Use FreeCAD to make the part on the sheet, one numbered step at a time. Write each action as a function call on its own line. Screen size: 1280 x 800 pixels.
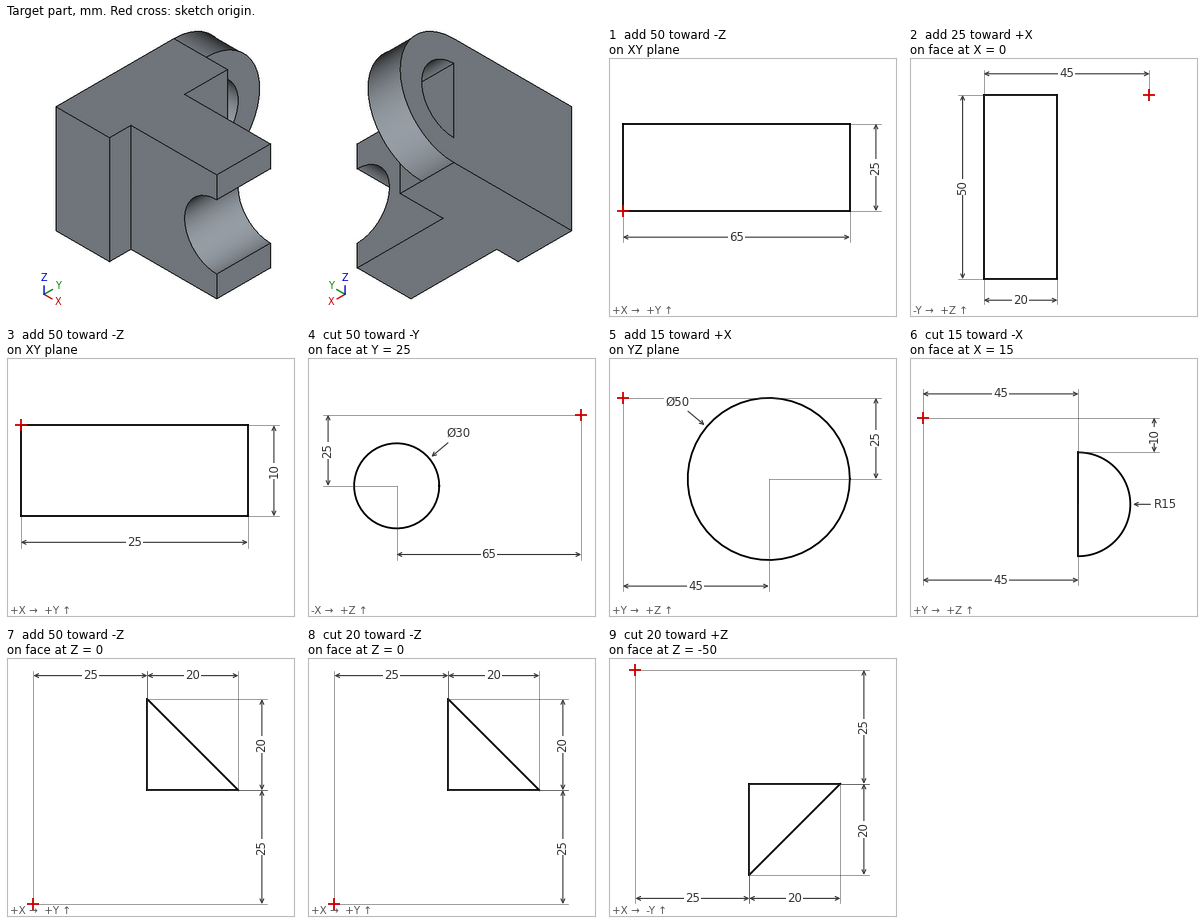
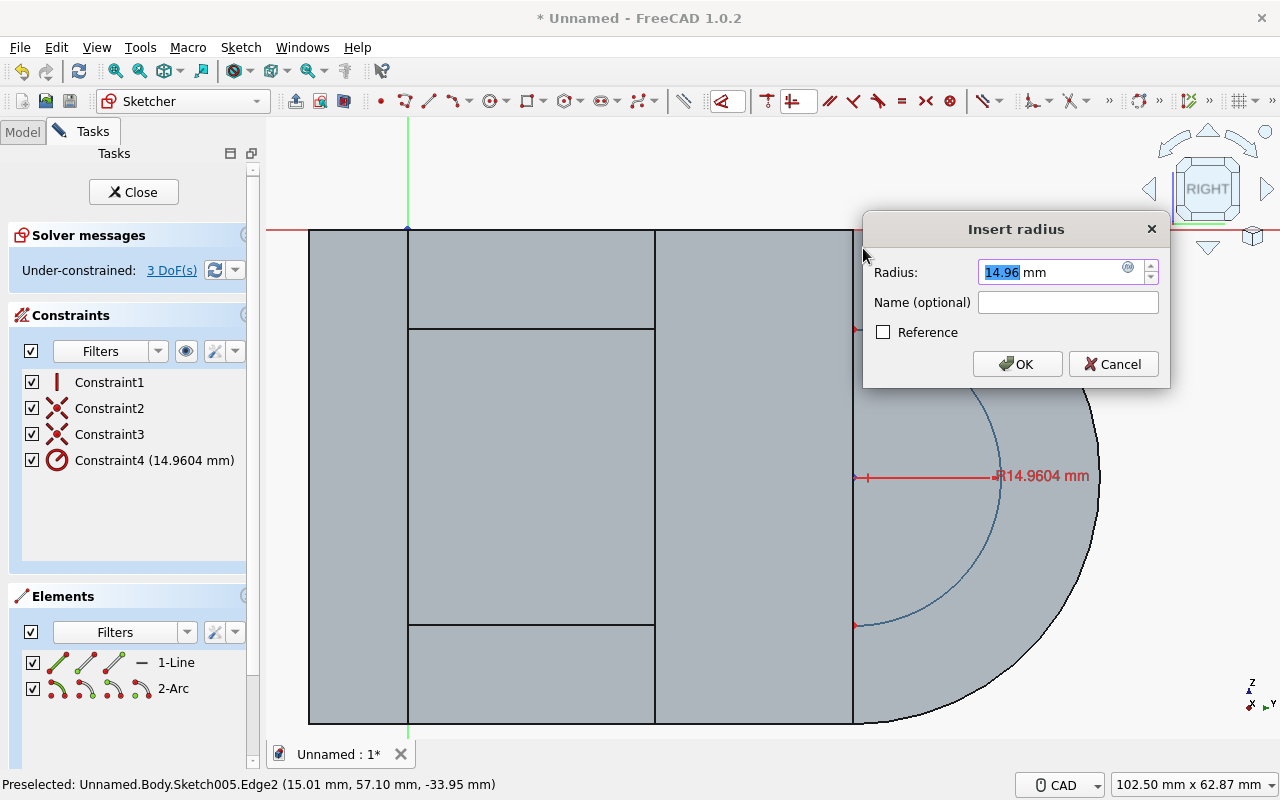
text(15)
key(Return)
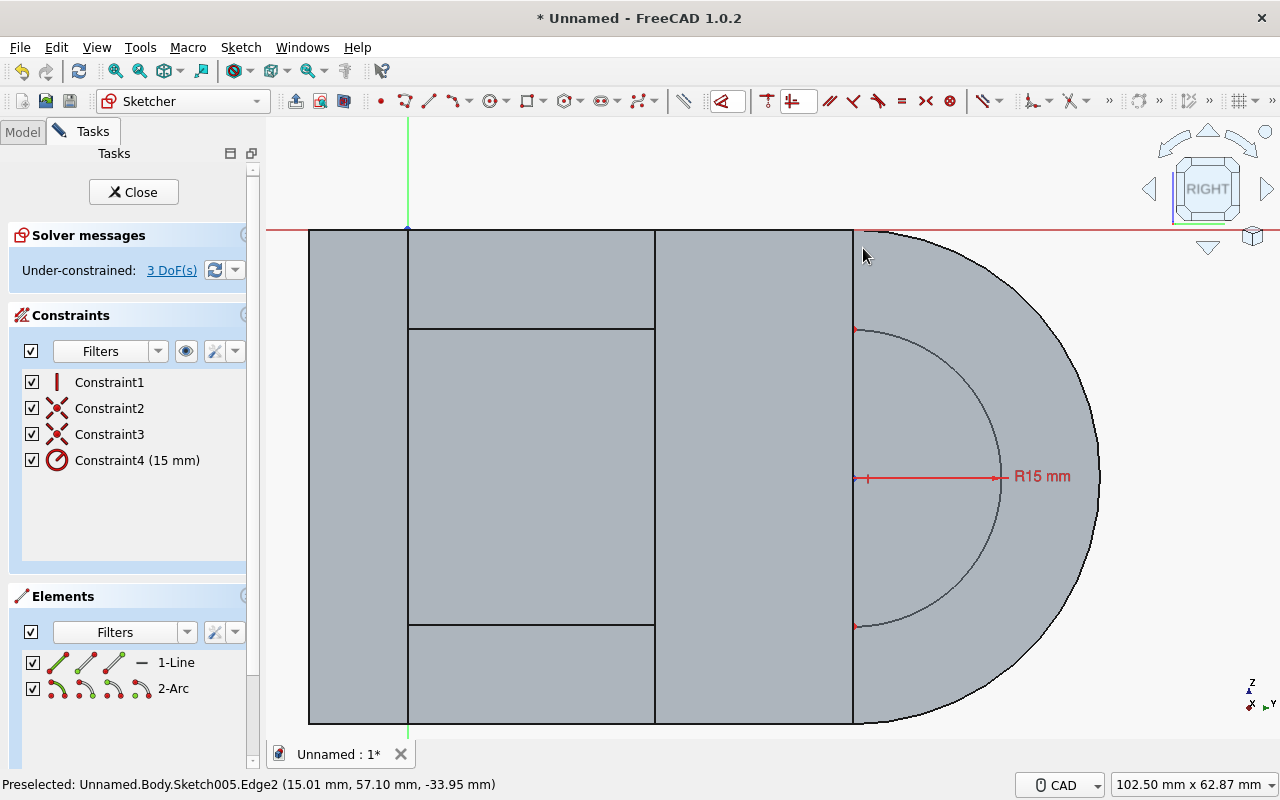
click(853, 330)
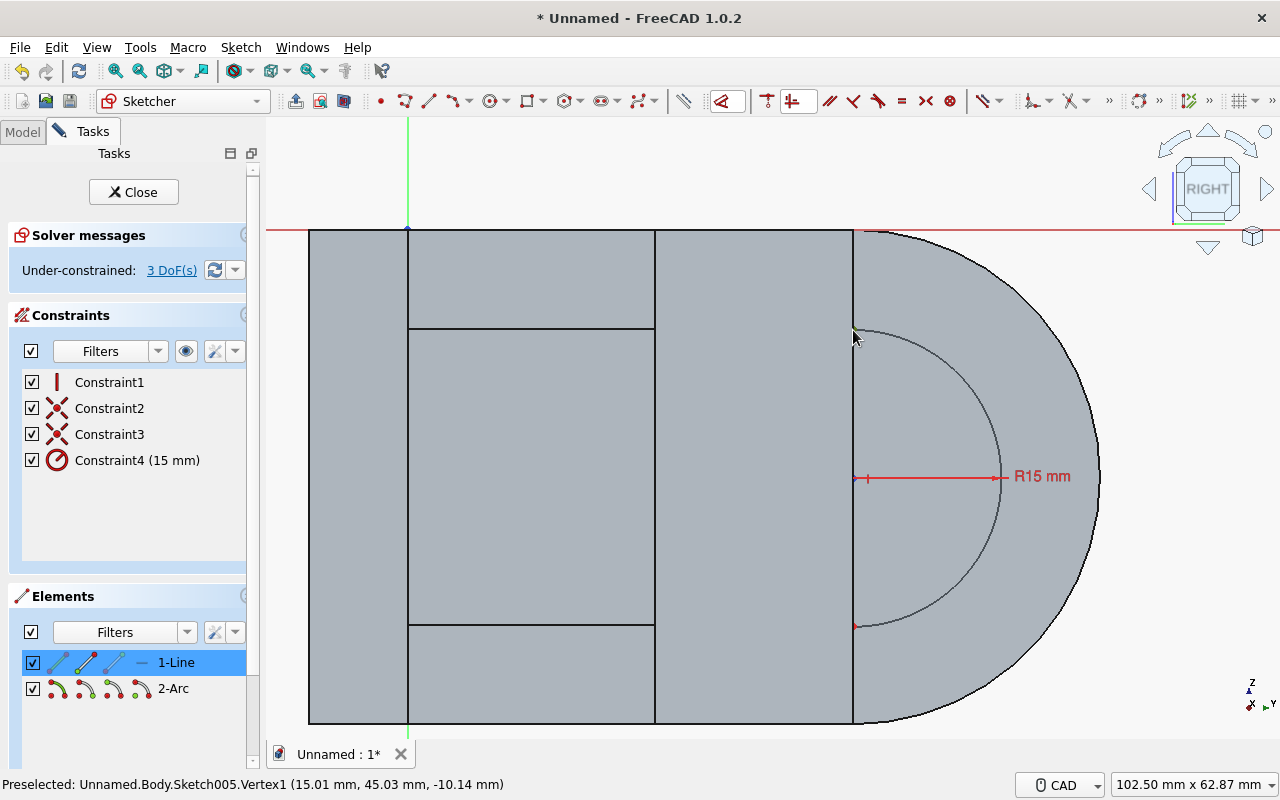
key(l)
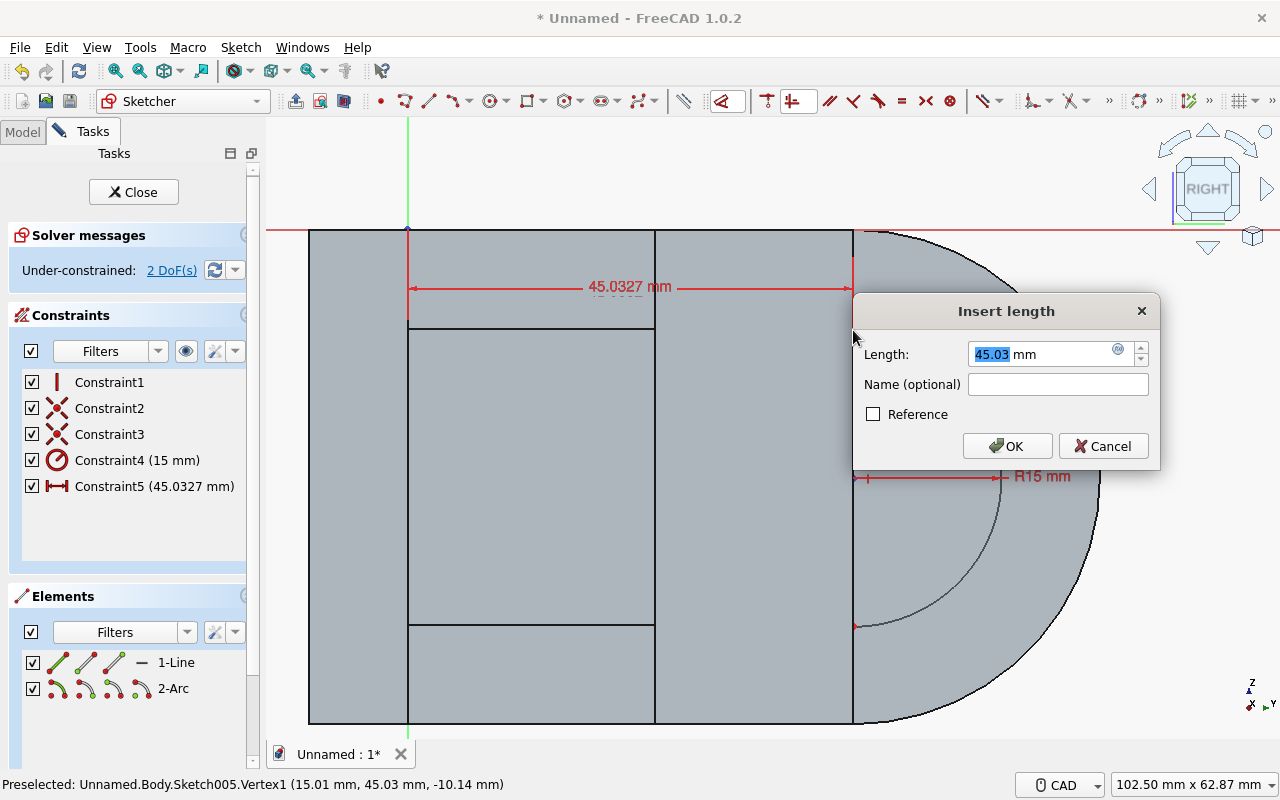
text(45)
key(Return)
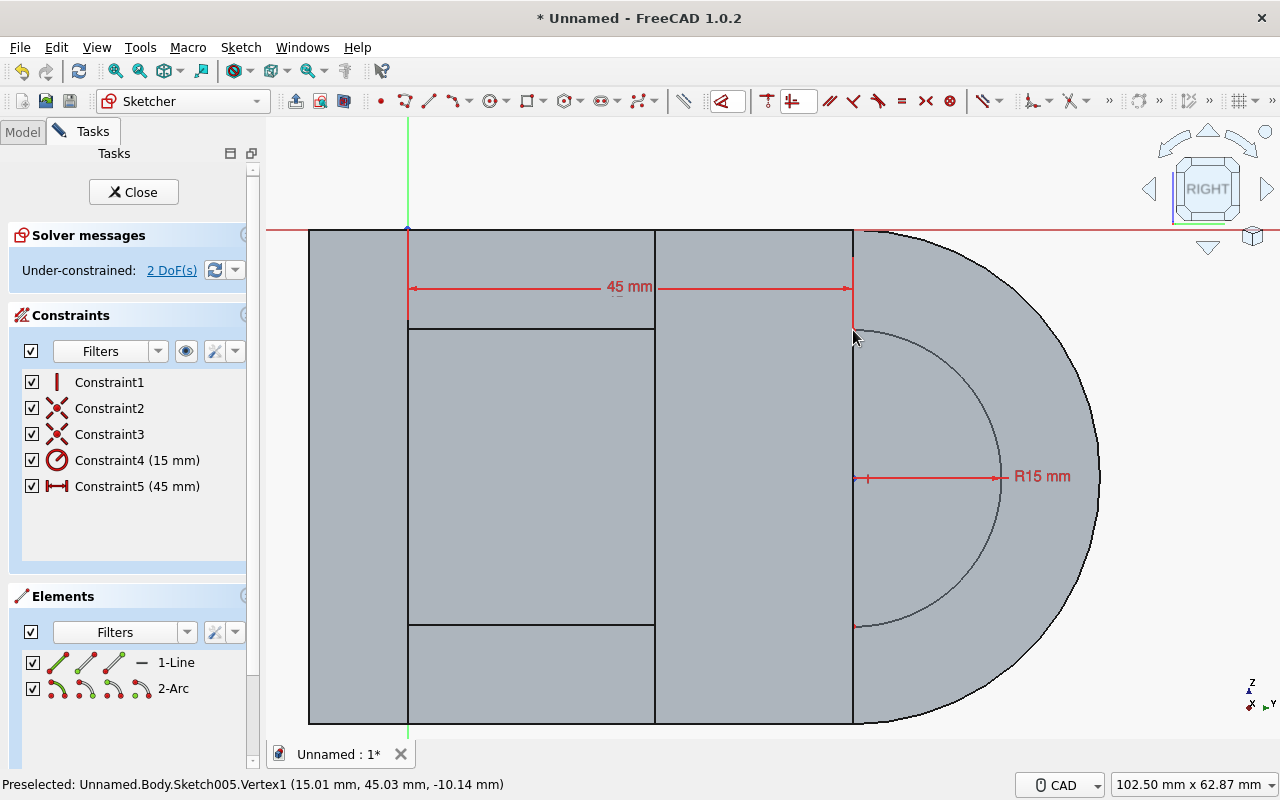
click(853, 330)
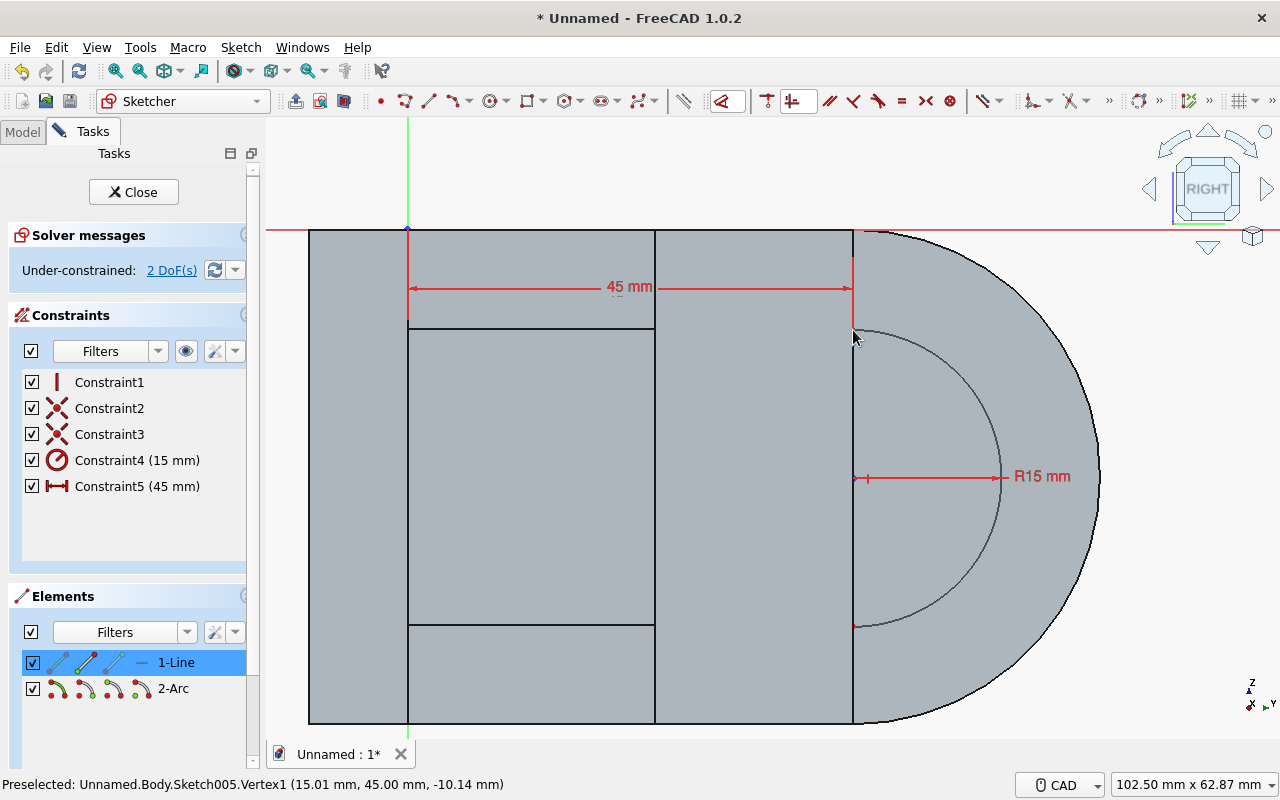
click(740, 102)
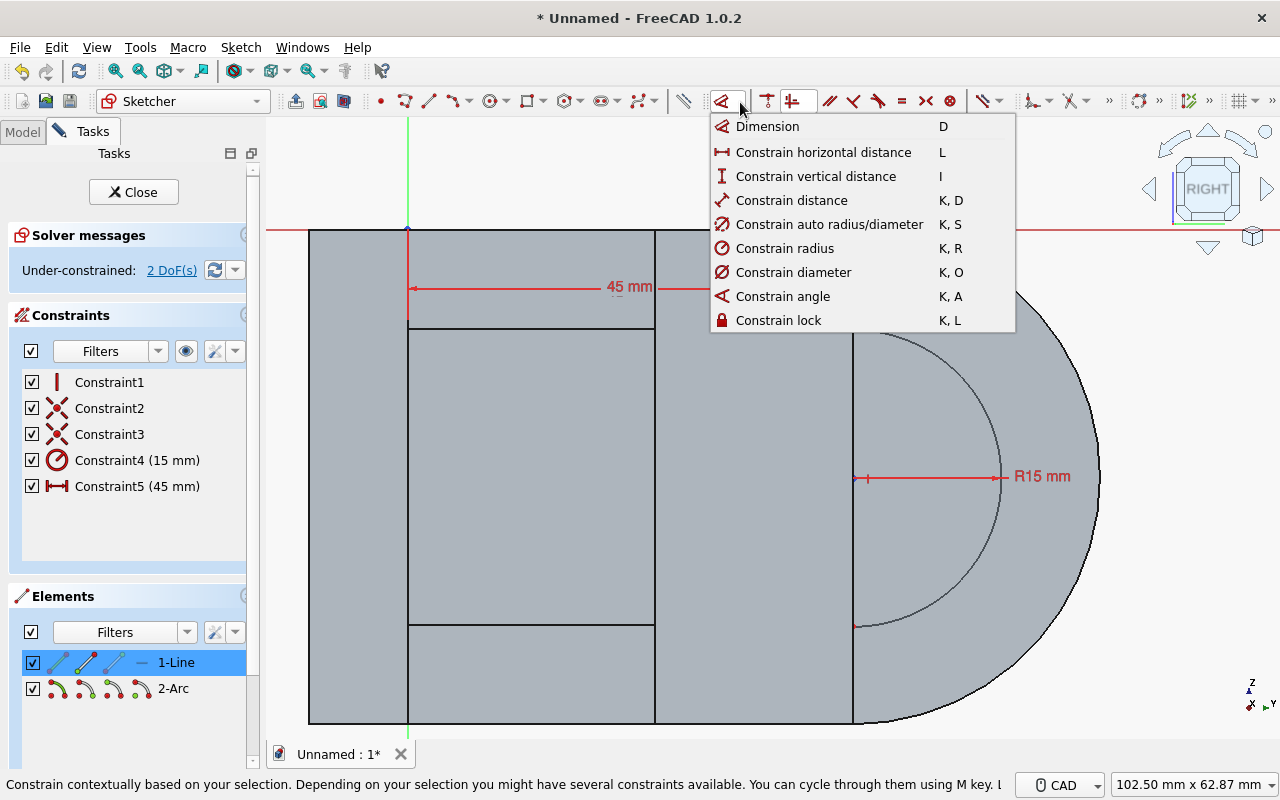
click(863, 176)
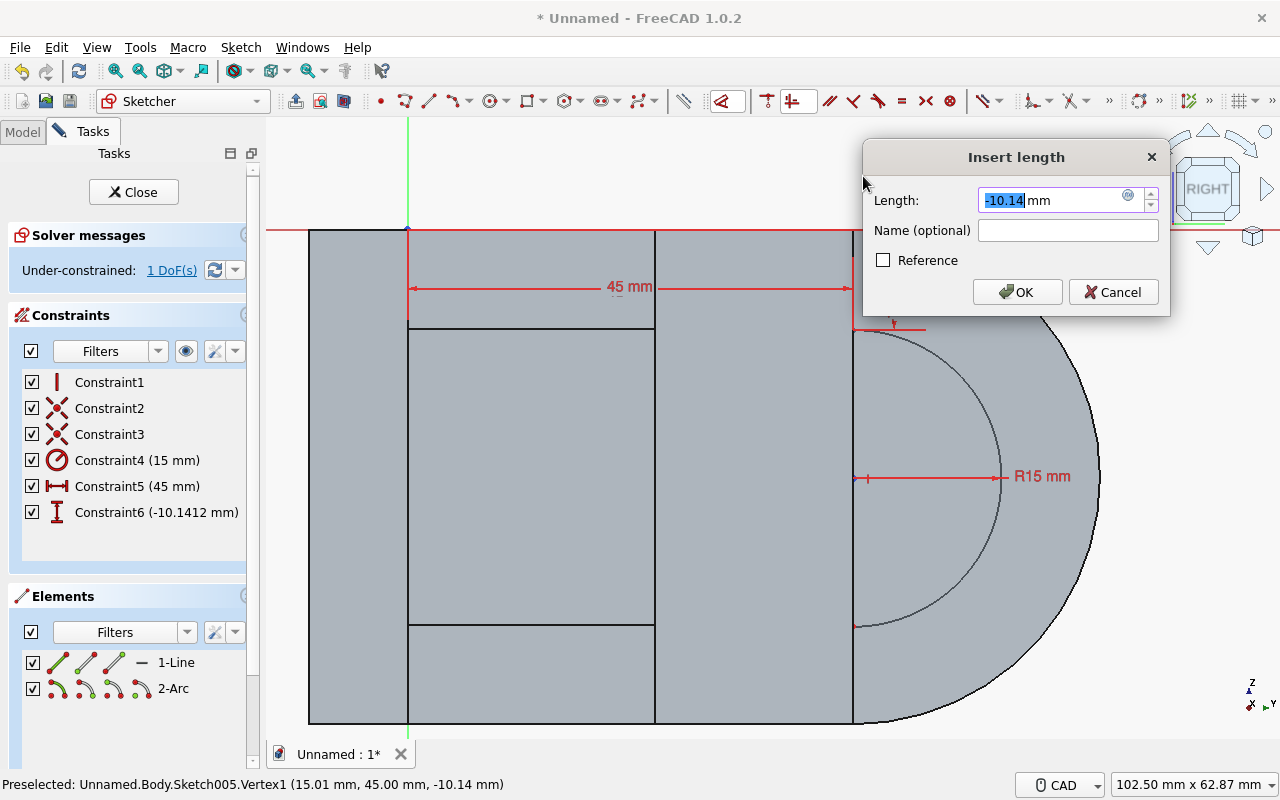
text(-10)
key(Return)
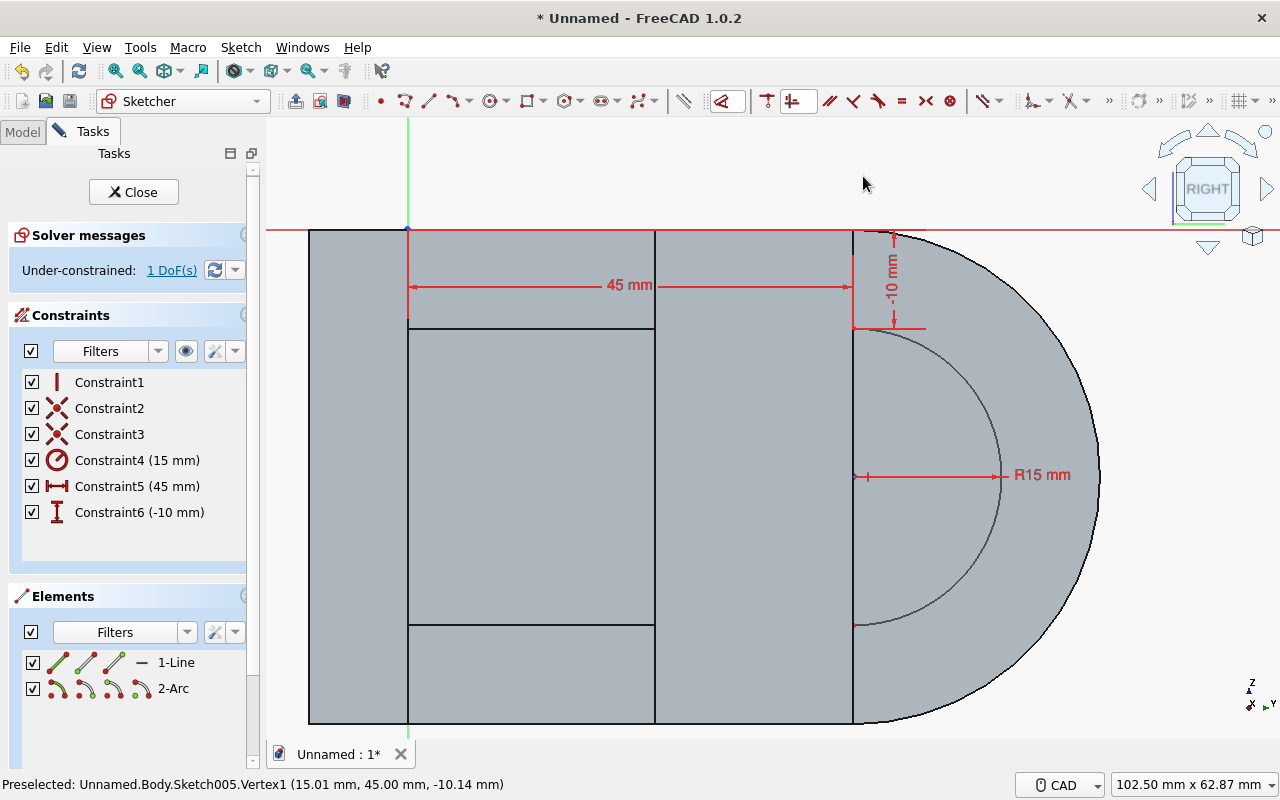
click(853, 477)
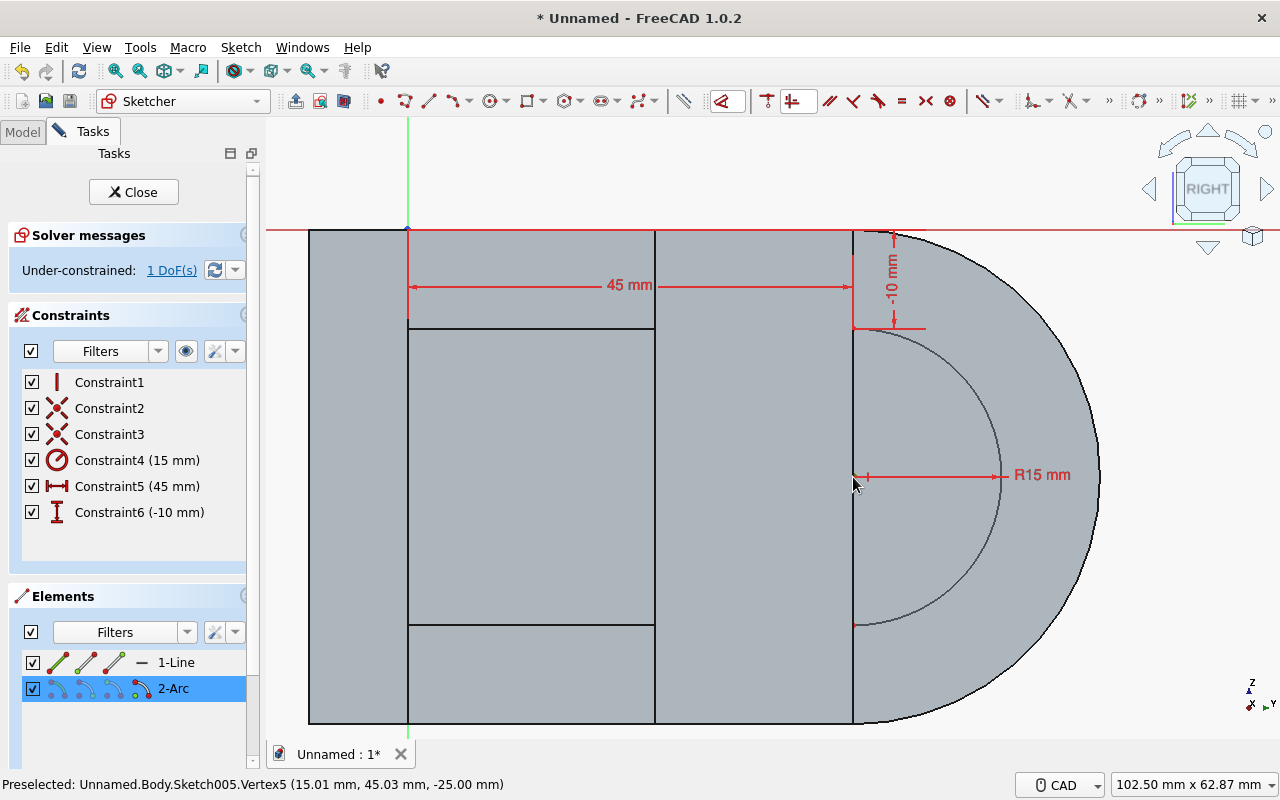
click(740, 102)